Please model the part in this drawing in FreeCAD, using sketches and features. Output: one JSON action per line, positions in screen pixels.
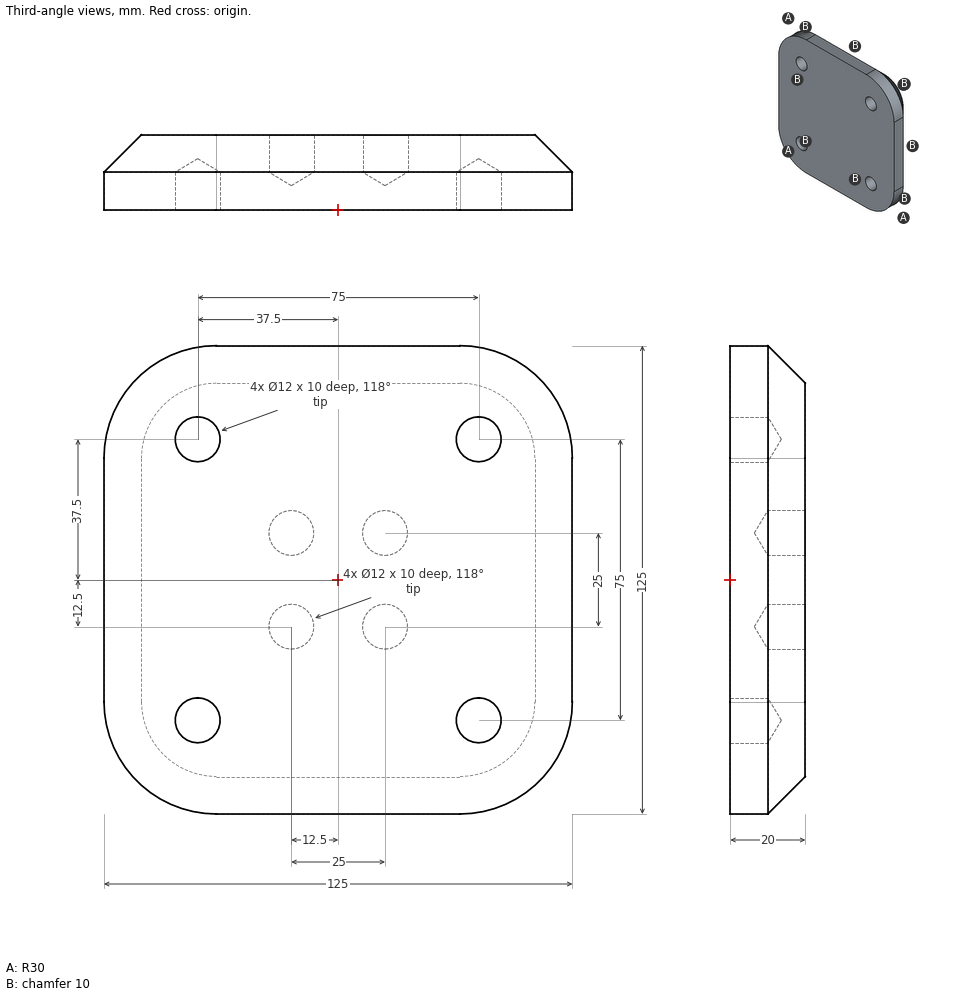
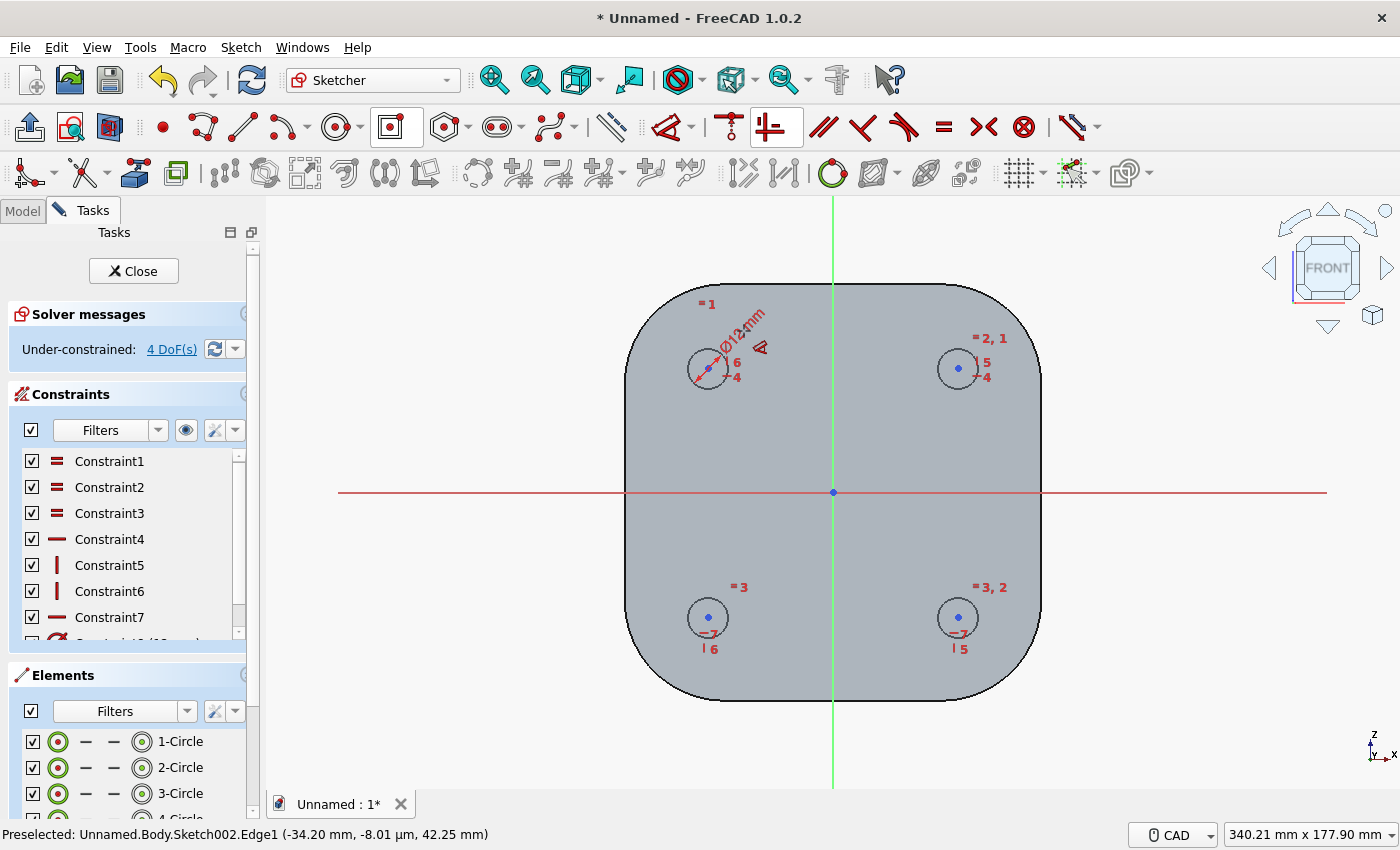
{"action": "left_click", "coordinate": [708, 369]}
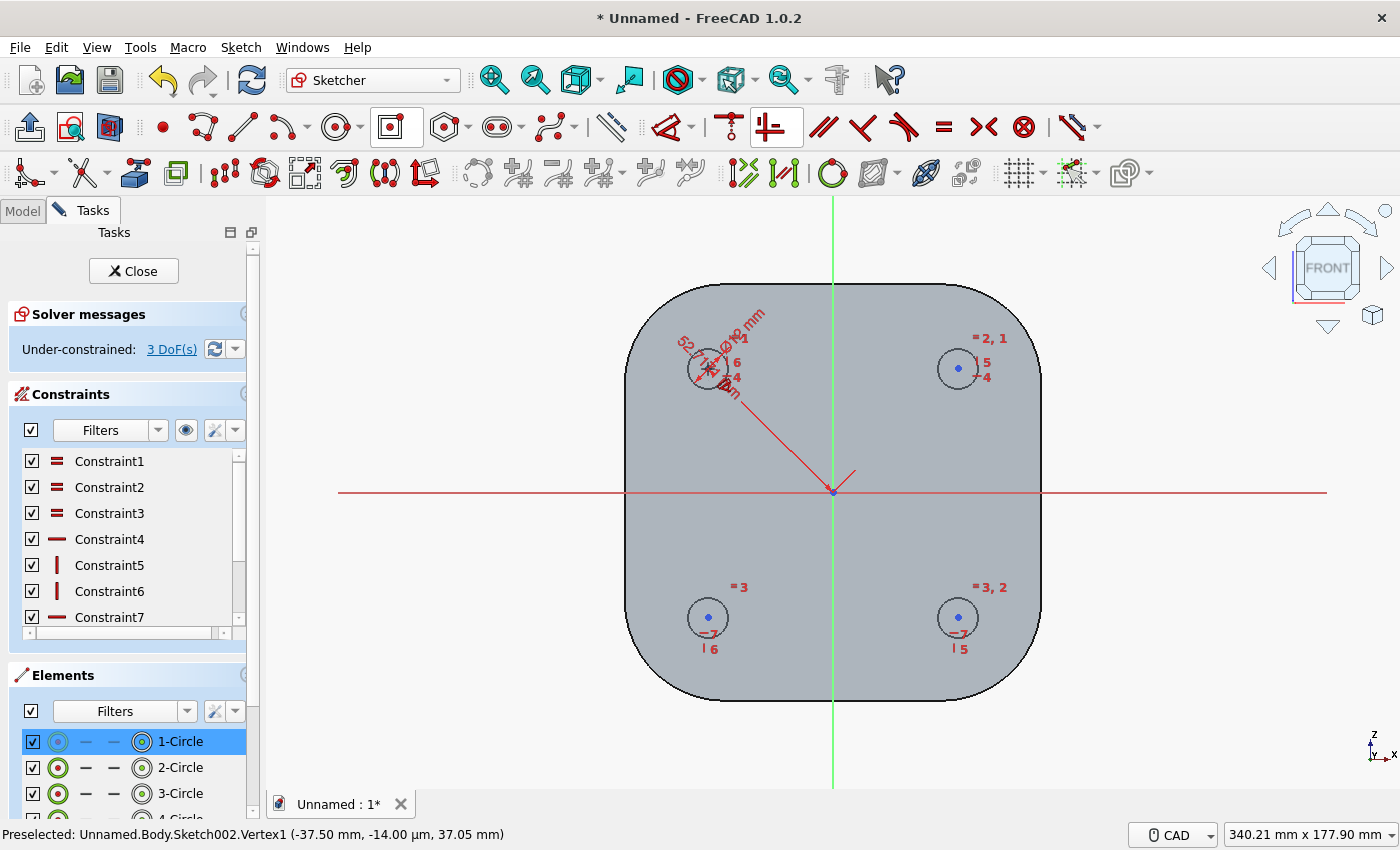
{"action": "left_click", "coordinate": [958, 369]}
{"action": "left_click", "coordinate": [890, 335]}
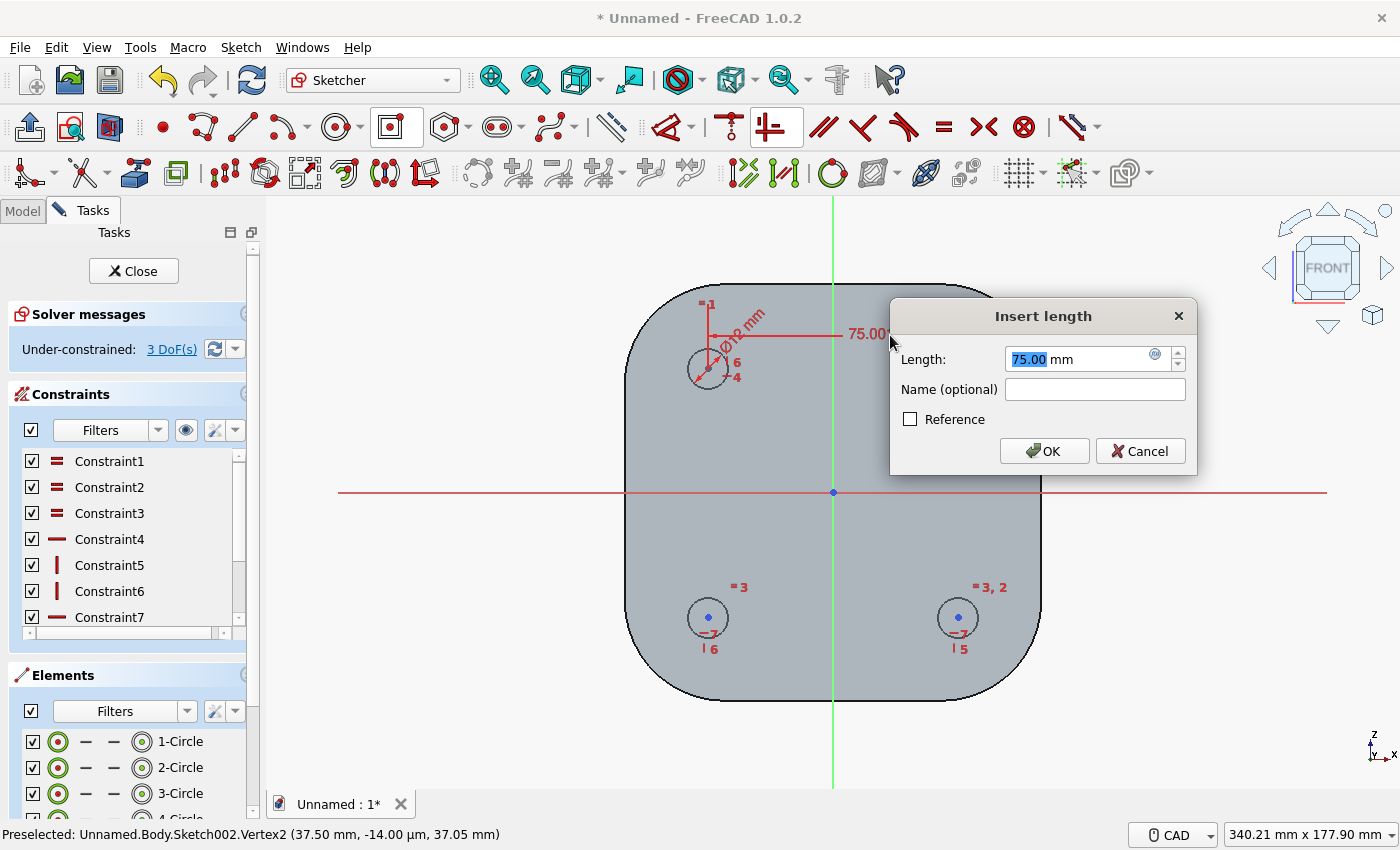
{"action": "type", "text": "75"}
{"action": "key", "text": "Return"}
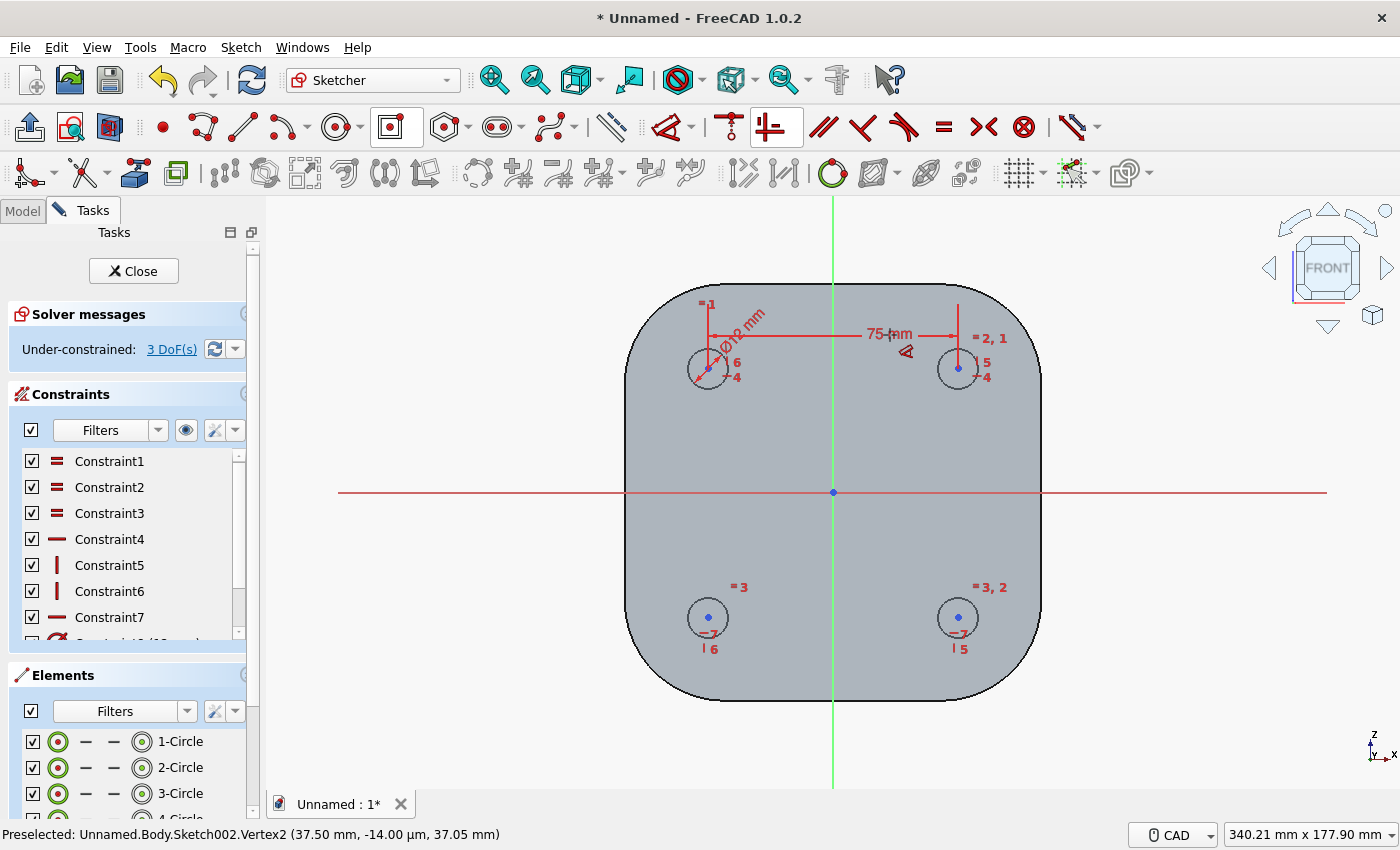
{"action": "left_click", "coordinate": [958, 369]}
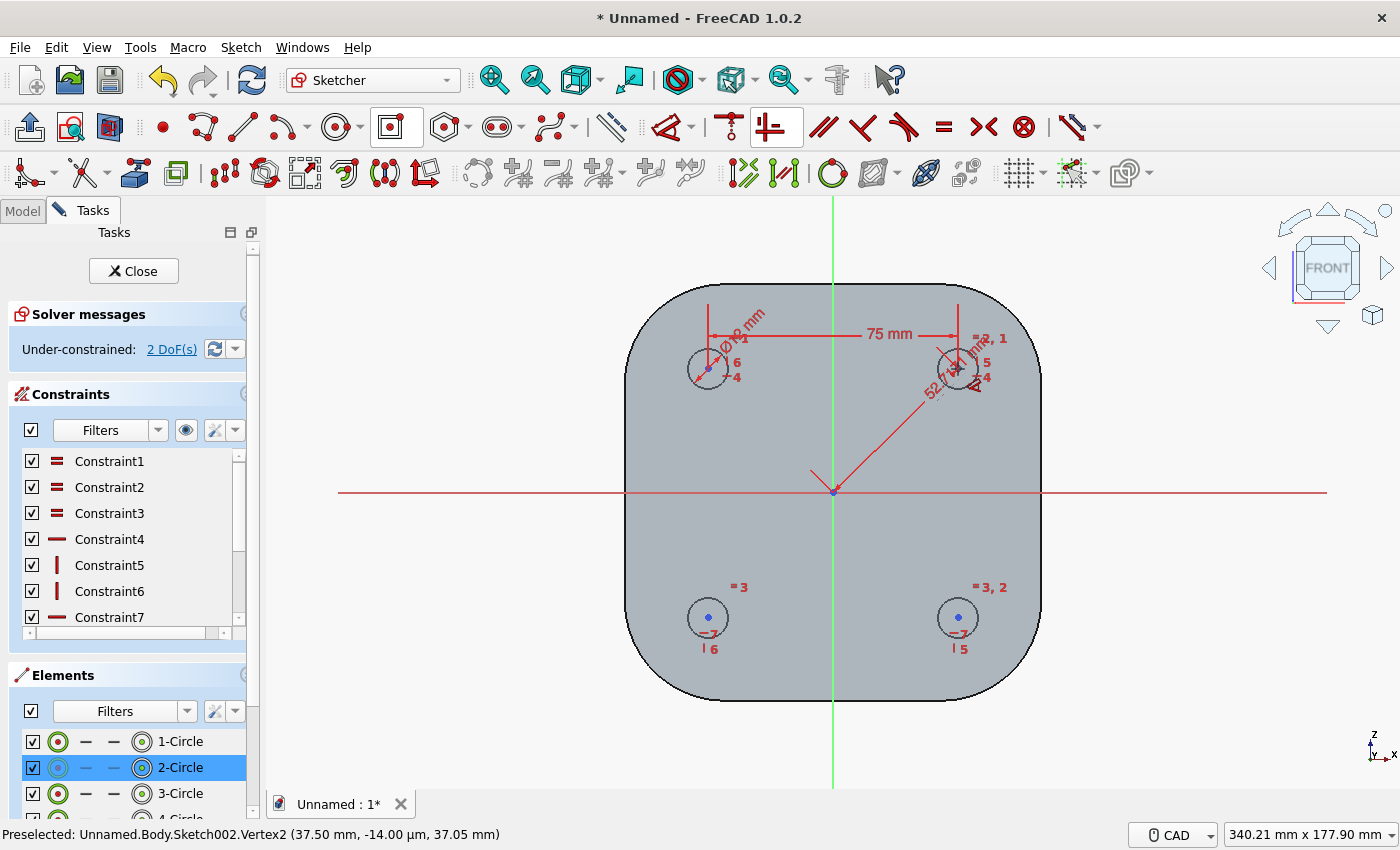
{"action": "left_click", "coordinate": [958, 618]}
{"action": "left_click", "coordinate": [992, 436]}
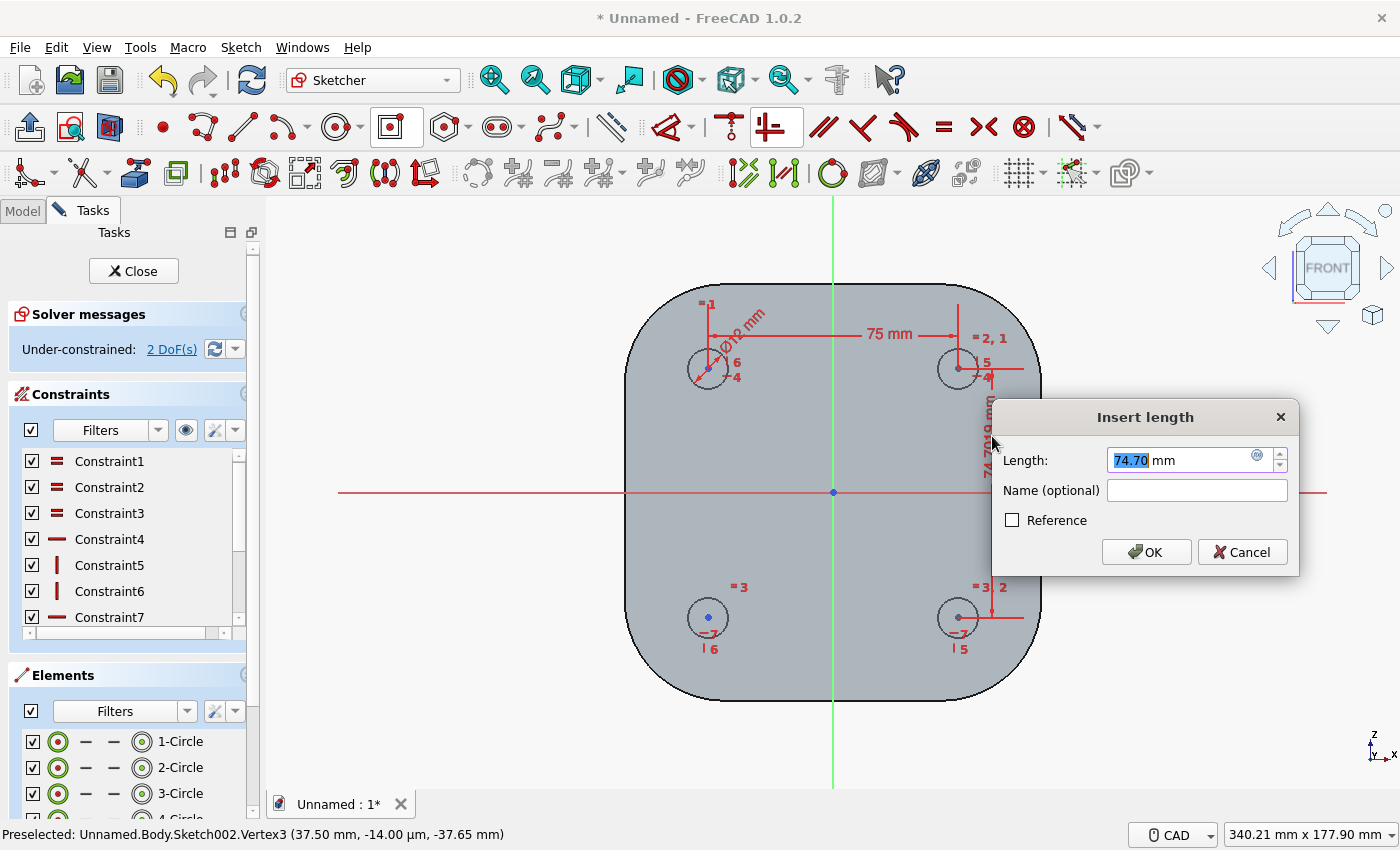
{"action": "type", "text": "75"}
{"action": "key", "text": "Return"}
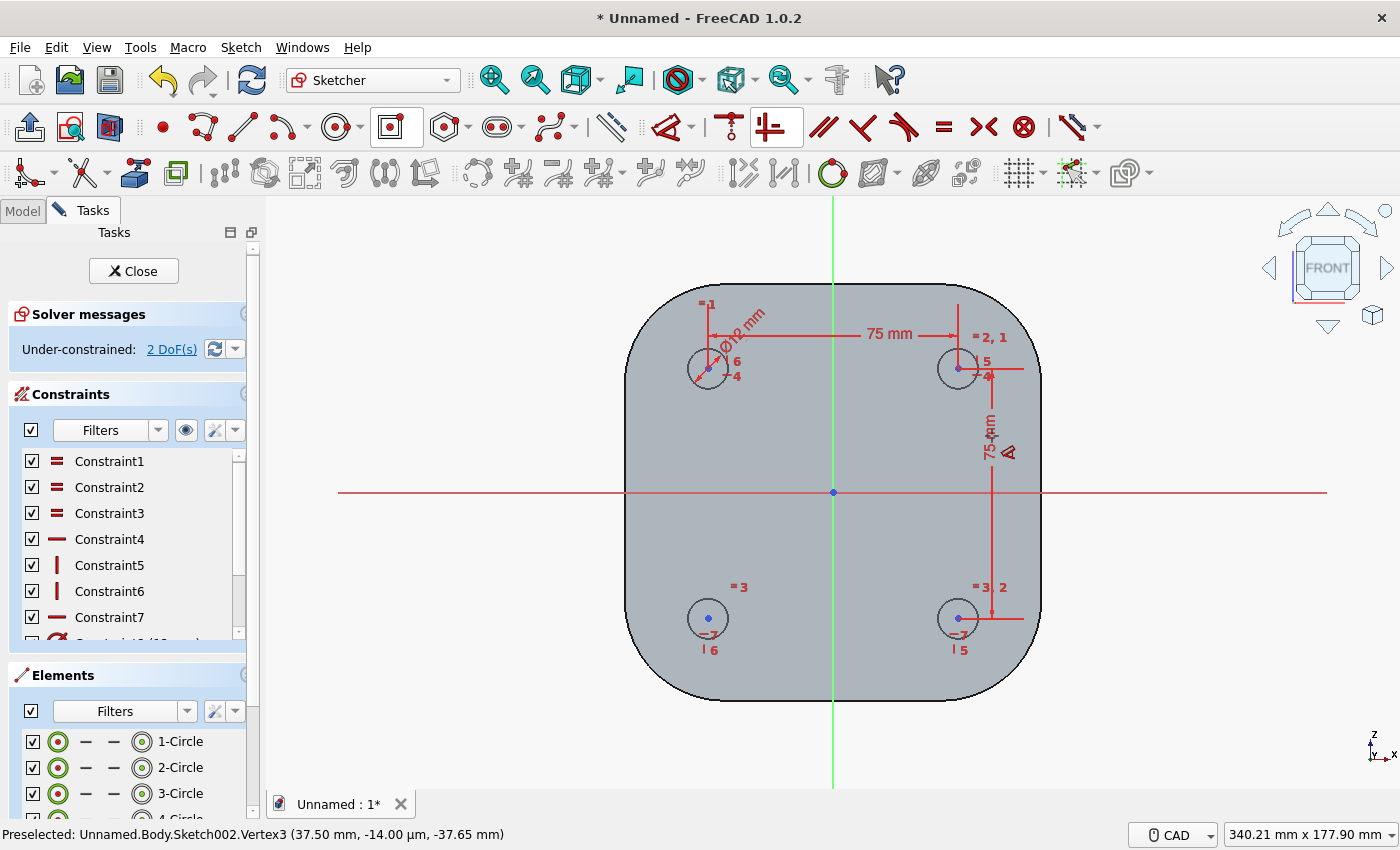
{"action": "left_click", "coordinate": [708, 369]}
{"action": "left_click", "coordinate": [814, 335]}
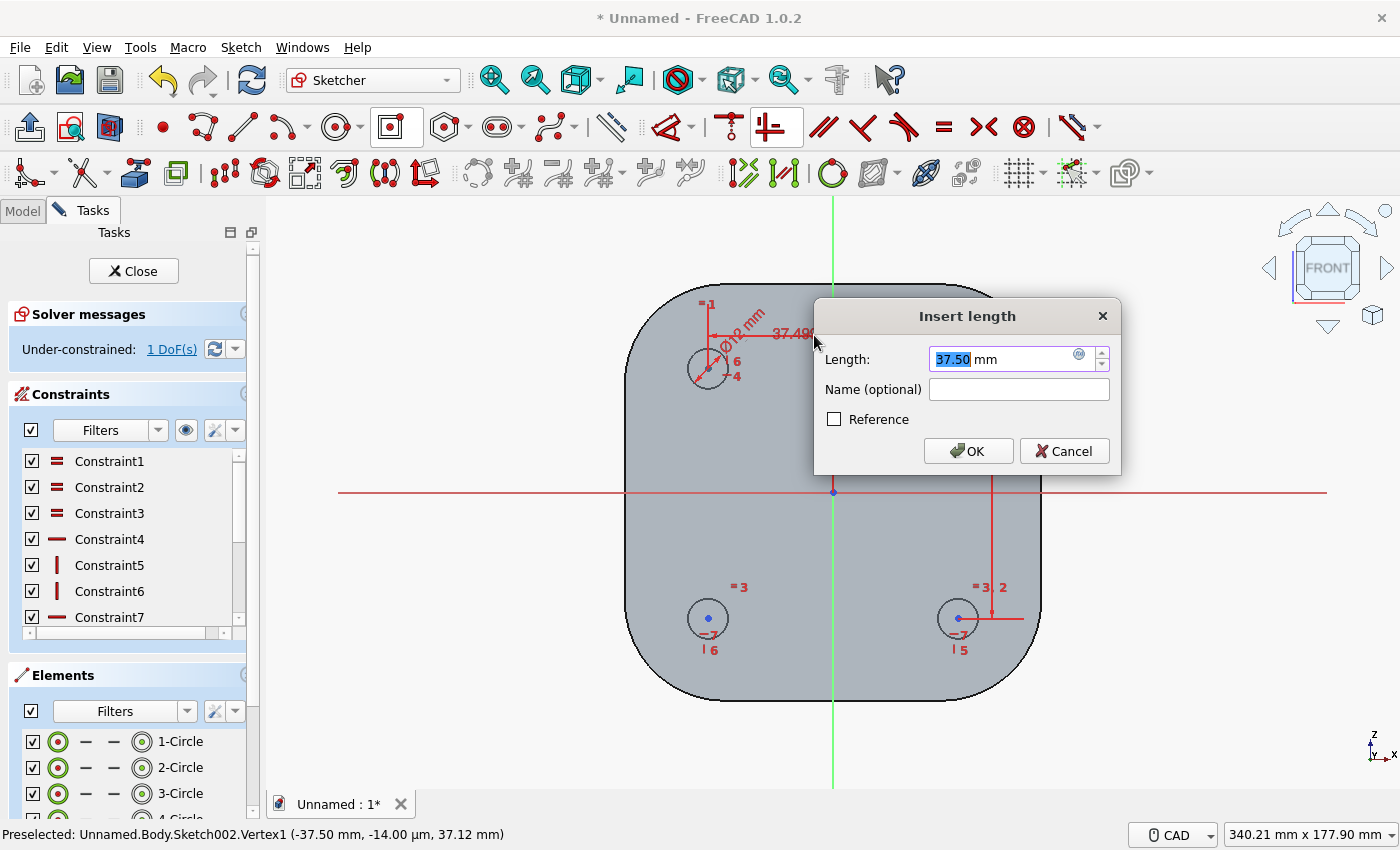
{"action": "type", "text": "37.5"}
{"action": "key", "text": "Return"}